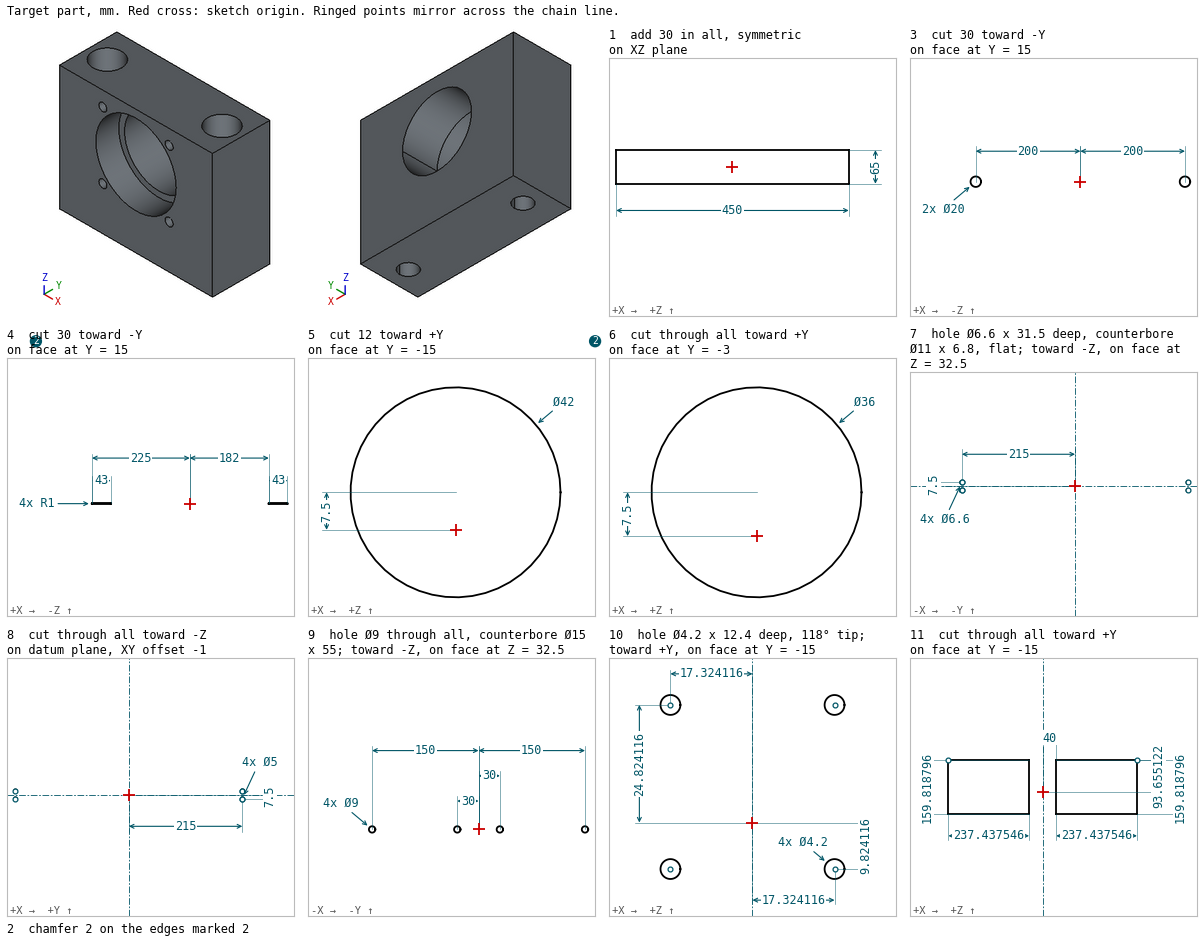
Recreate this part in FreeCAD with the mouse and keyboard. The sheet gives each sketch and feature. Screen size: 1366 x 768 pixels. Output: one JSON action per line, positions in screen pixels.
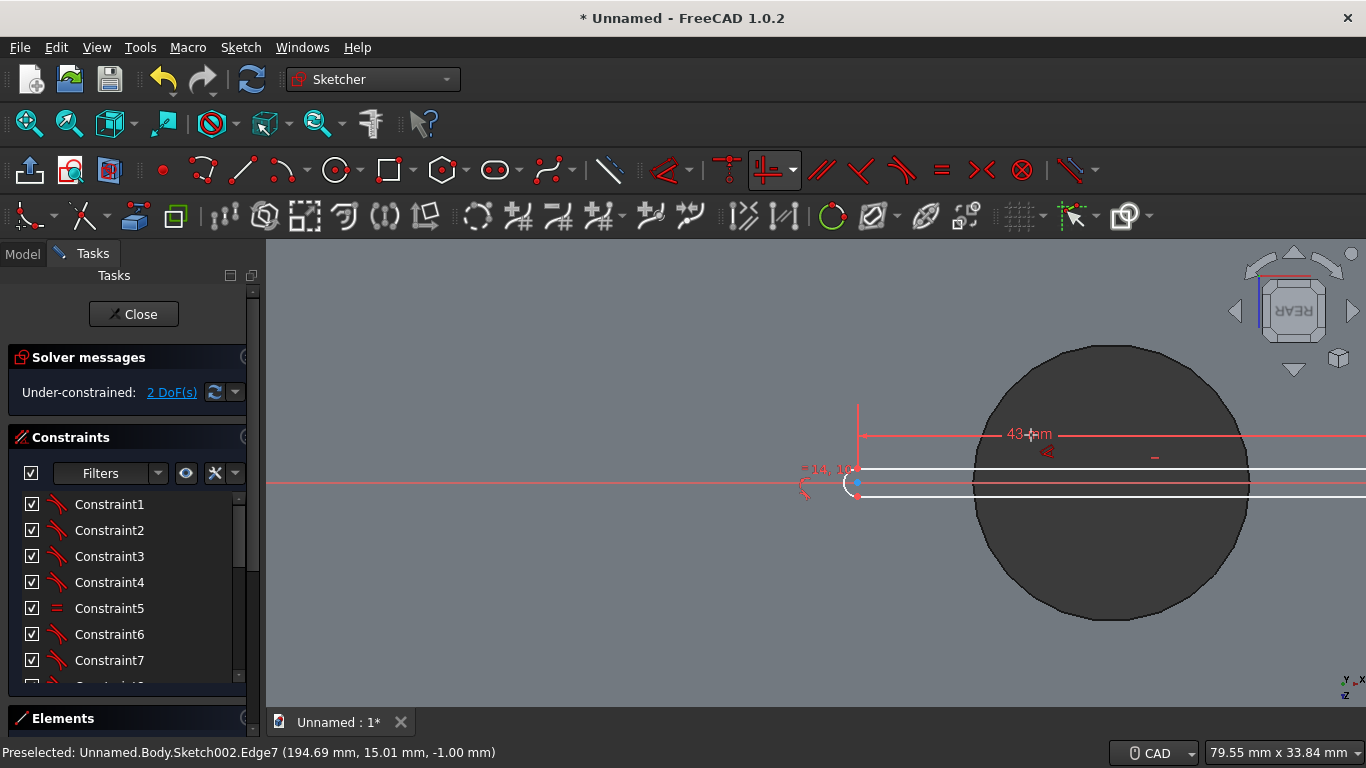
{"action": "scroll", "coordinate": [1047, 472], "scroll_direction": "down", "scroll_amount": 11}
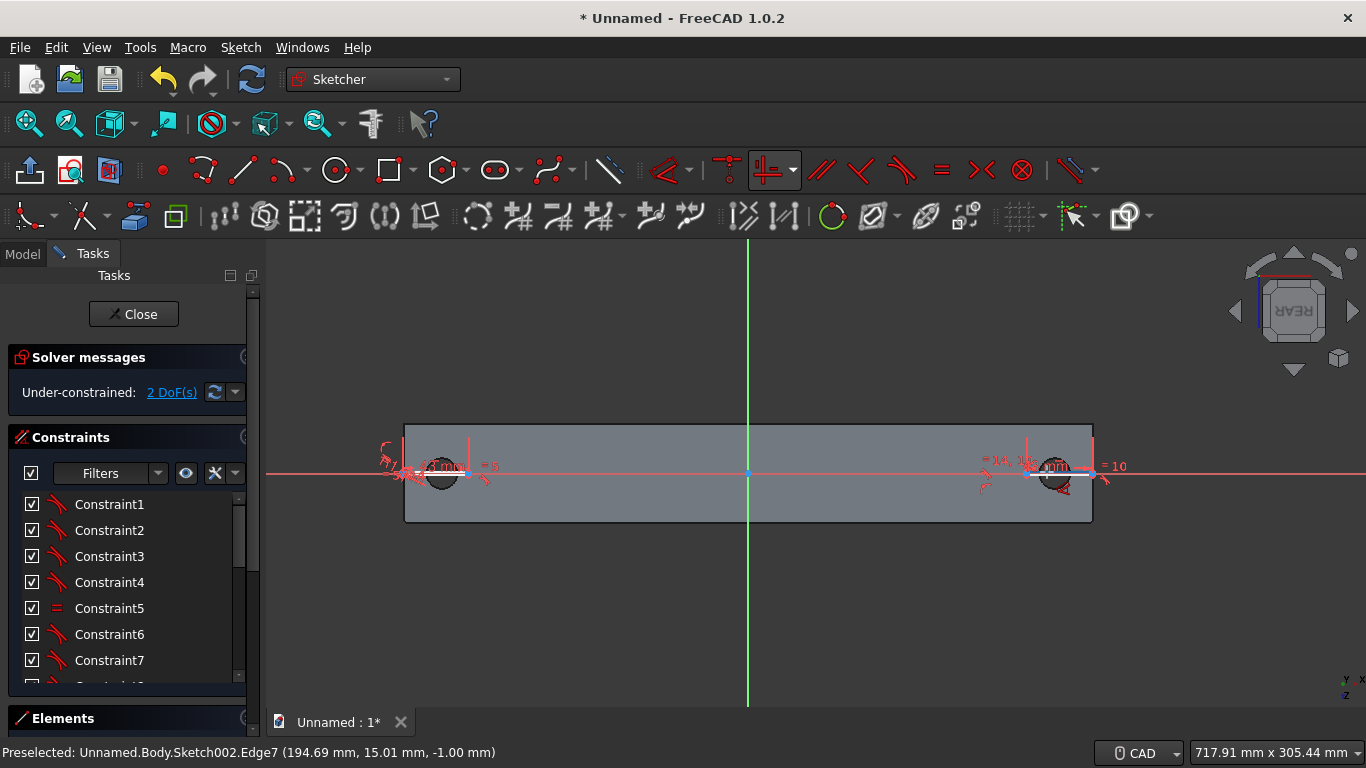
{"action": "scroll", "coordinate": [403, 472], "scroll_direction": "up", "scroll_amount": 11}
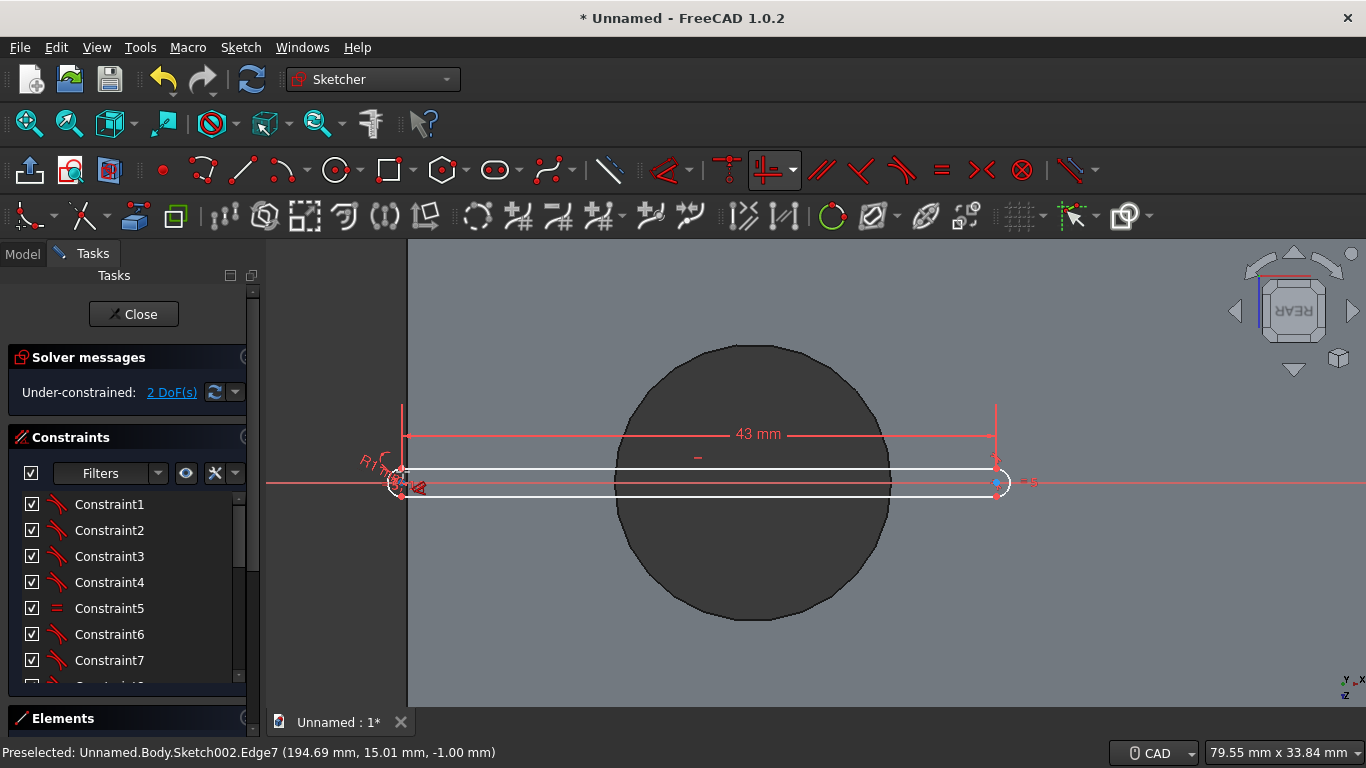
{"action": "left_click", "coordinate": [402, 469]}
{"action": "left_click", "coordinate": [617, 435]}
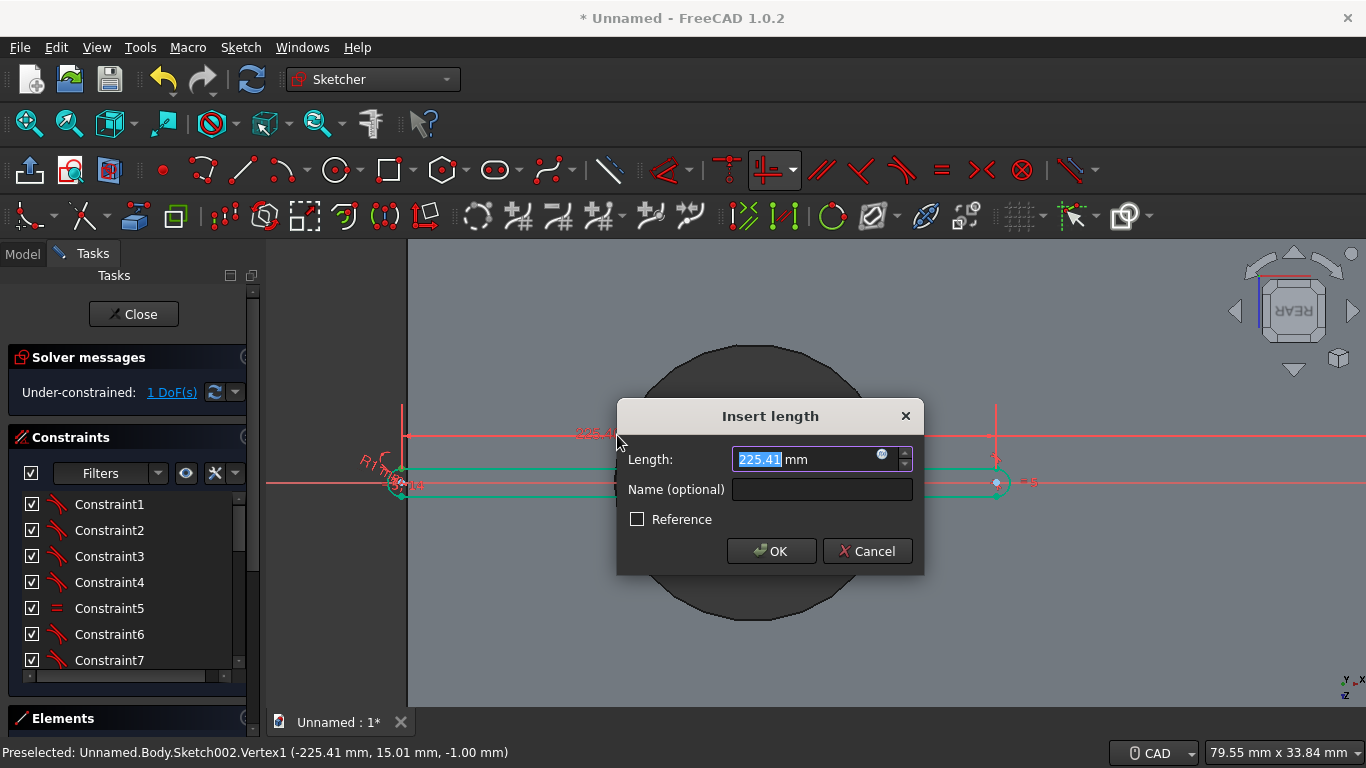
{"action": "type", "text": "225"}
{"action": "key", "text": "Return"}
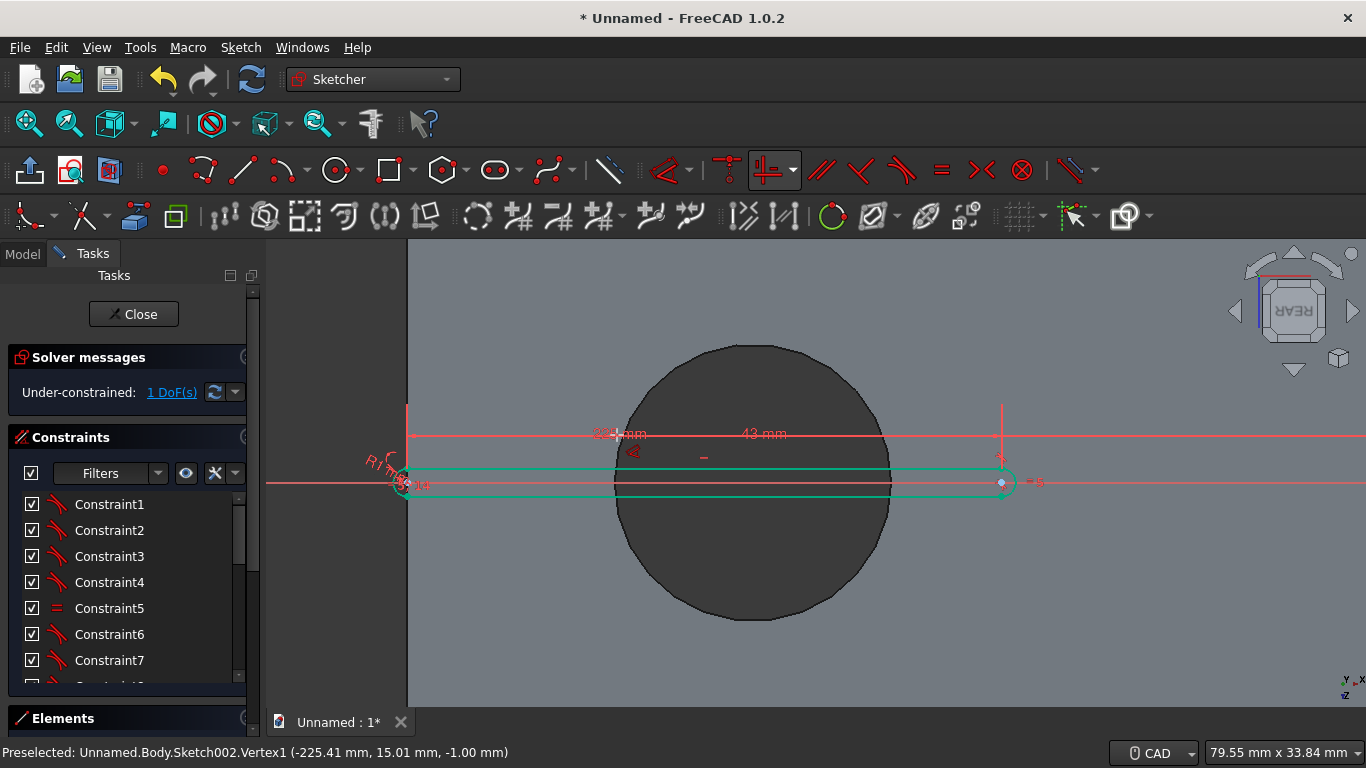
{"action": "scroll", "coordinate": [402, 472], "scroll_direction": "down", "scroll_amount": 11}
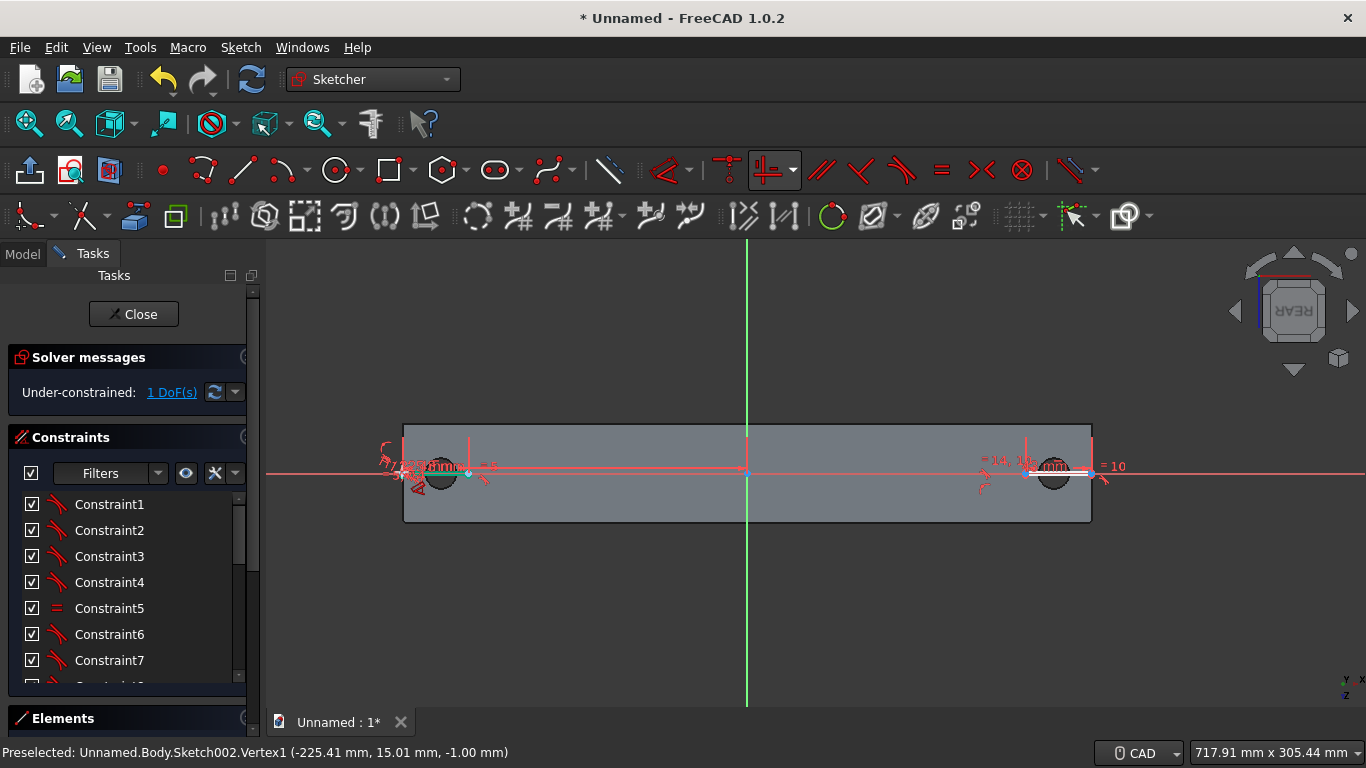
{"action": "scroll", "coordinate": [1026, 472], "scroll_direction": "up", "scroll_amount": 11}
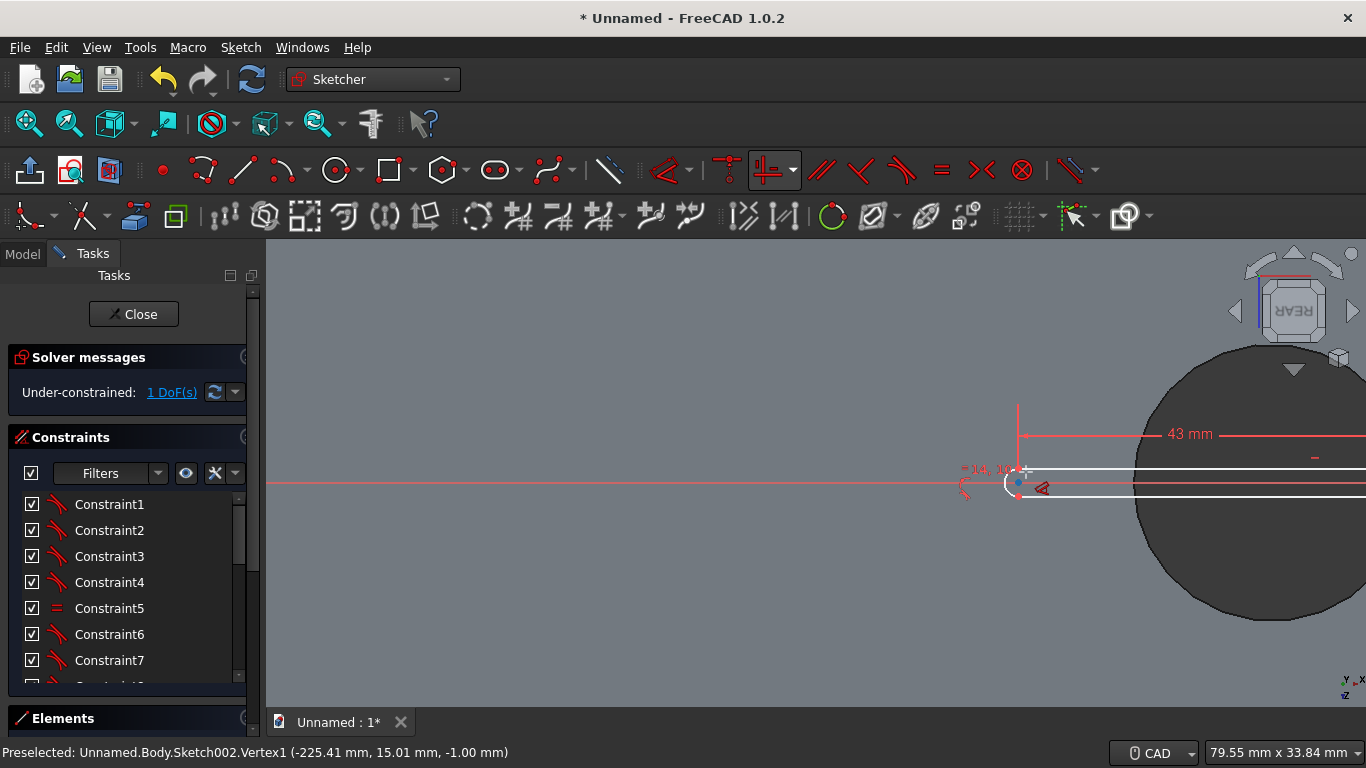
{"action": "left_click", "coordinate": [1018, 469]}
{"action": "left_click", "coordinate": [656, 435]}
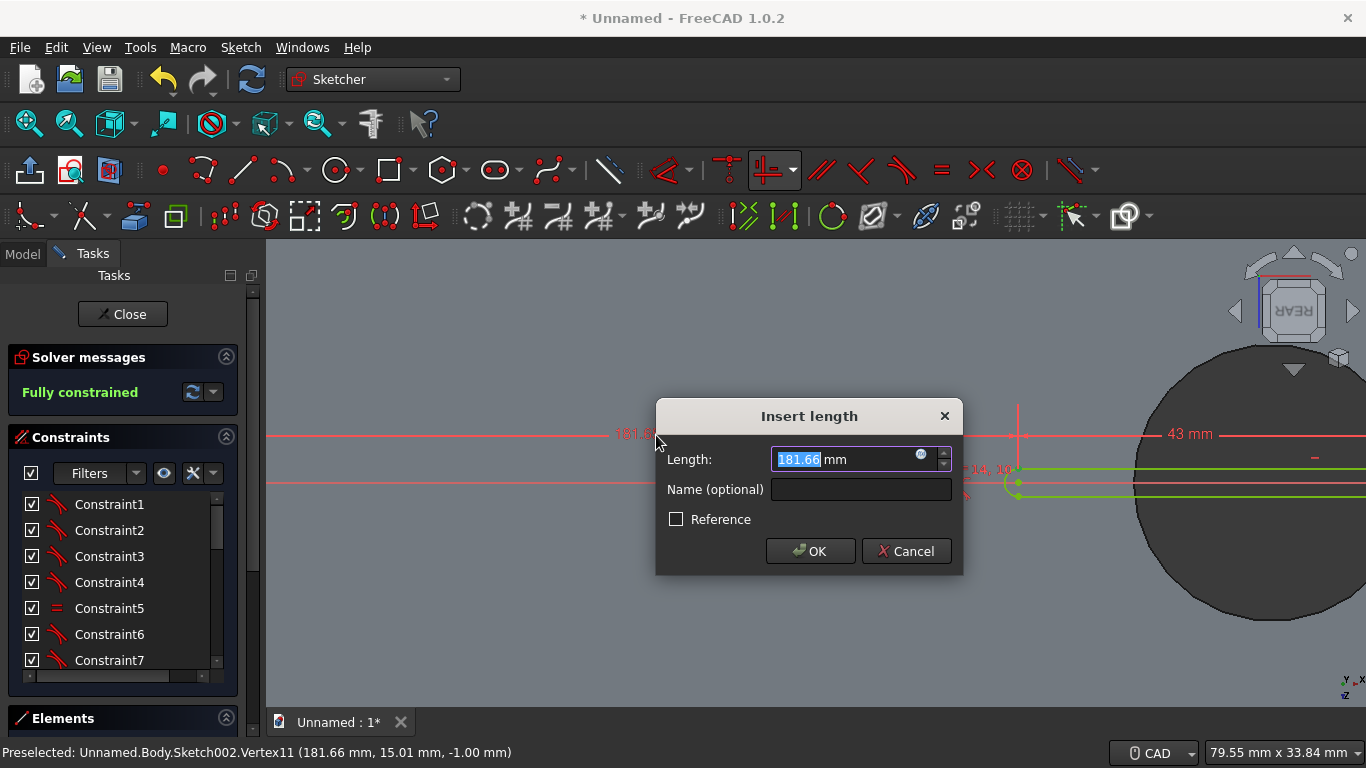
{"action": "type", "text": "182"}
{"action": "key", "text": "Return"}
{"action": "key", "text": "Escape"}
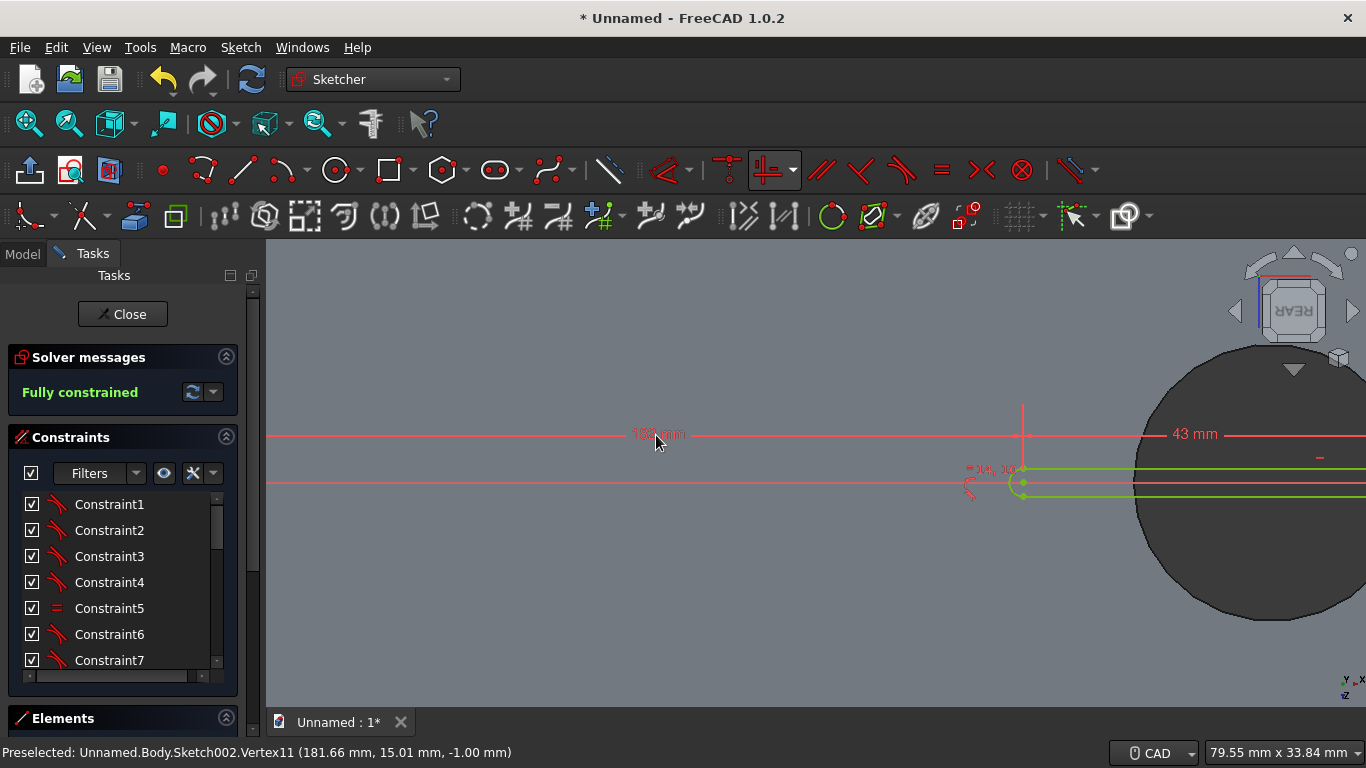
{"action": "left_click", "coordinate": [123, 314]}